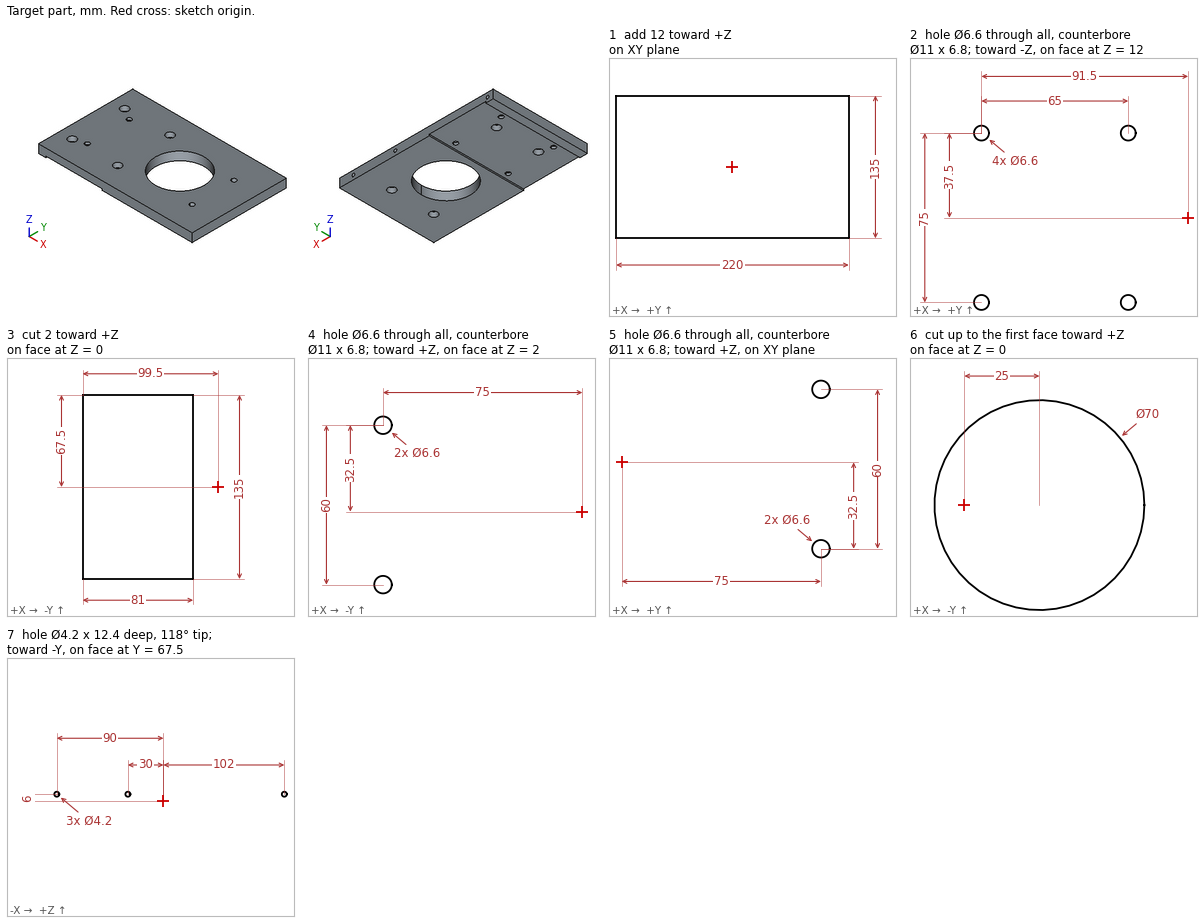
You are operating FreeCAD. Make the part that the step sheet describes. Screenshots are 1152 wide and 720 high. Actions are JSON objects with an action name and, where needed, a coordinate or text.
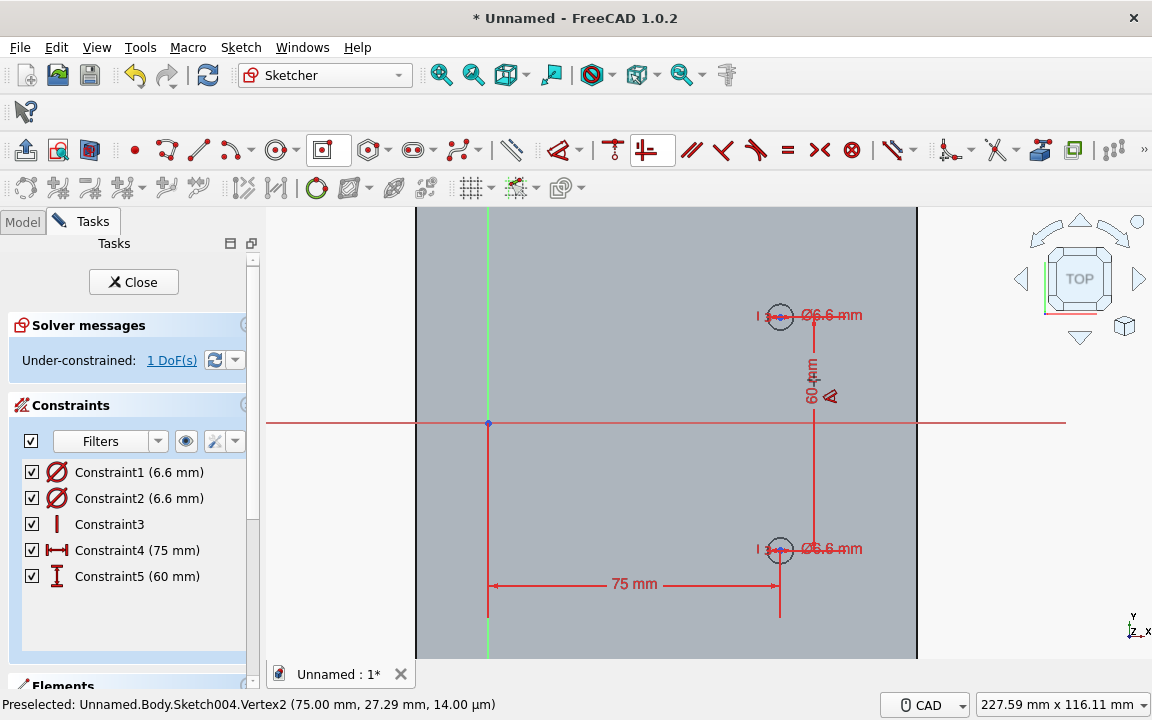
{"action": "left_click", "coordinate": [780, 551]}
{"action": "left_click", "coordinate": [454, 487]}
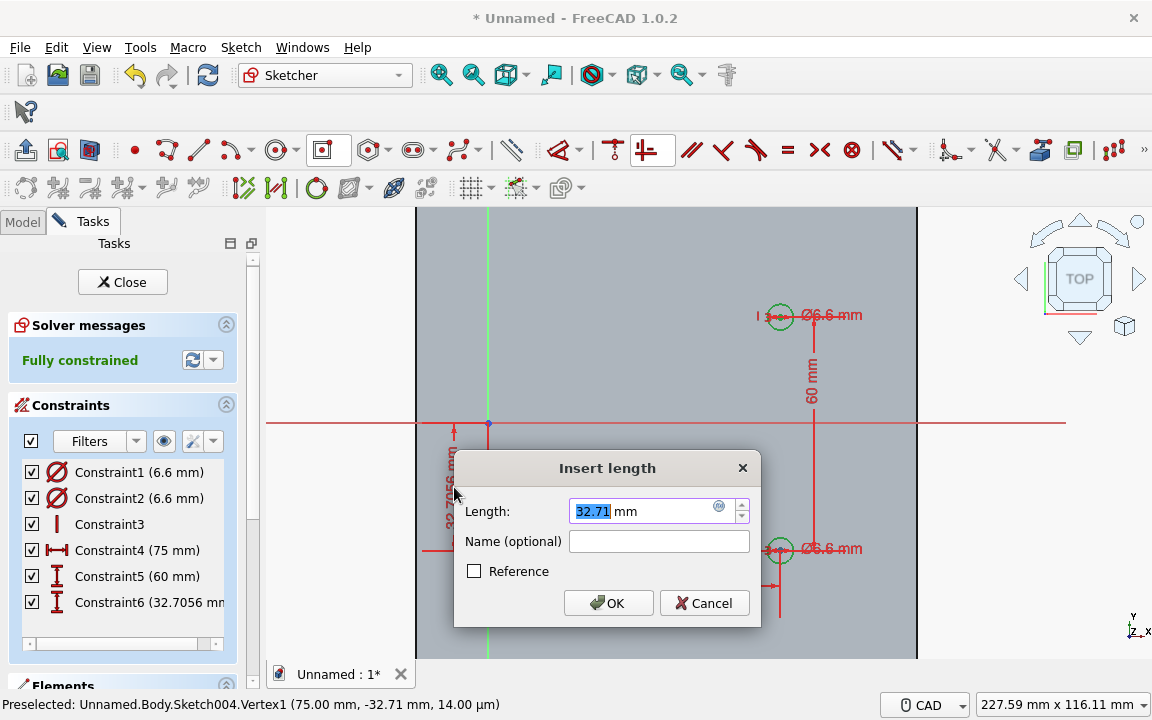
{"action": "type", "text": "32.5"}
{"action": "key", "text": "Return"}
{"action": "key", "text": "Escape"}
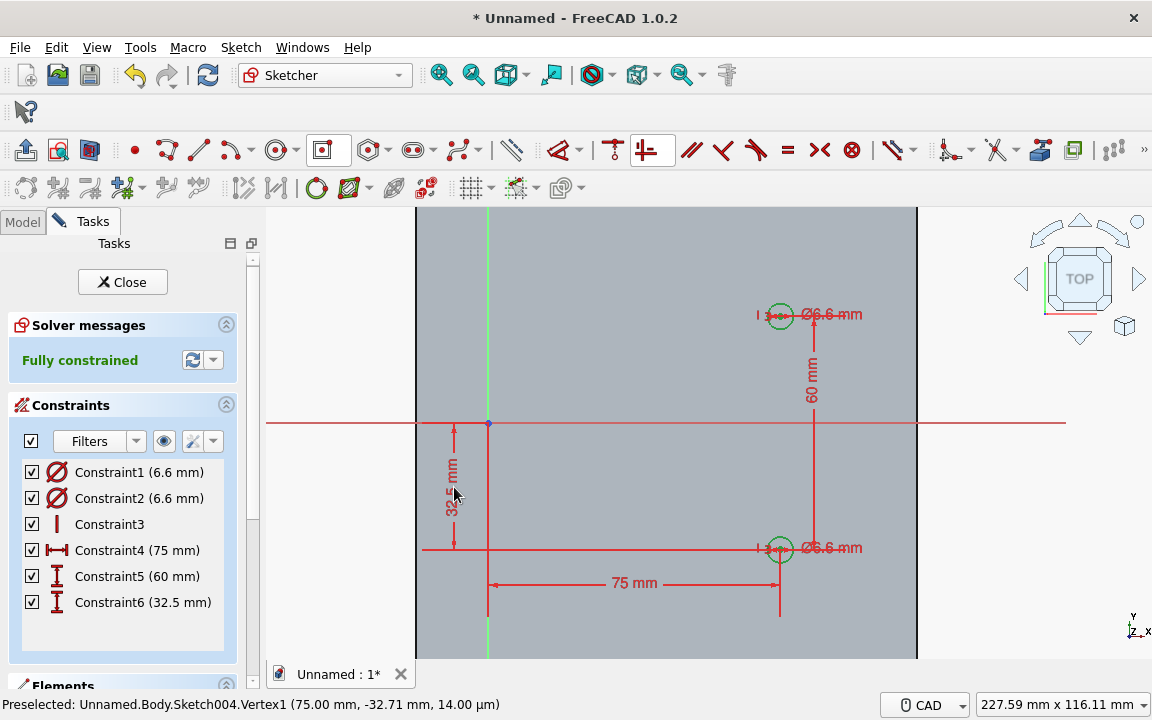
{"action": "left_click", "coordinate": [123, 282]}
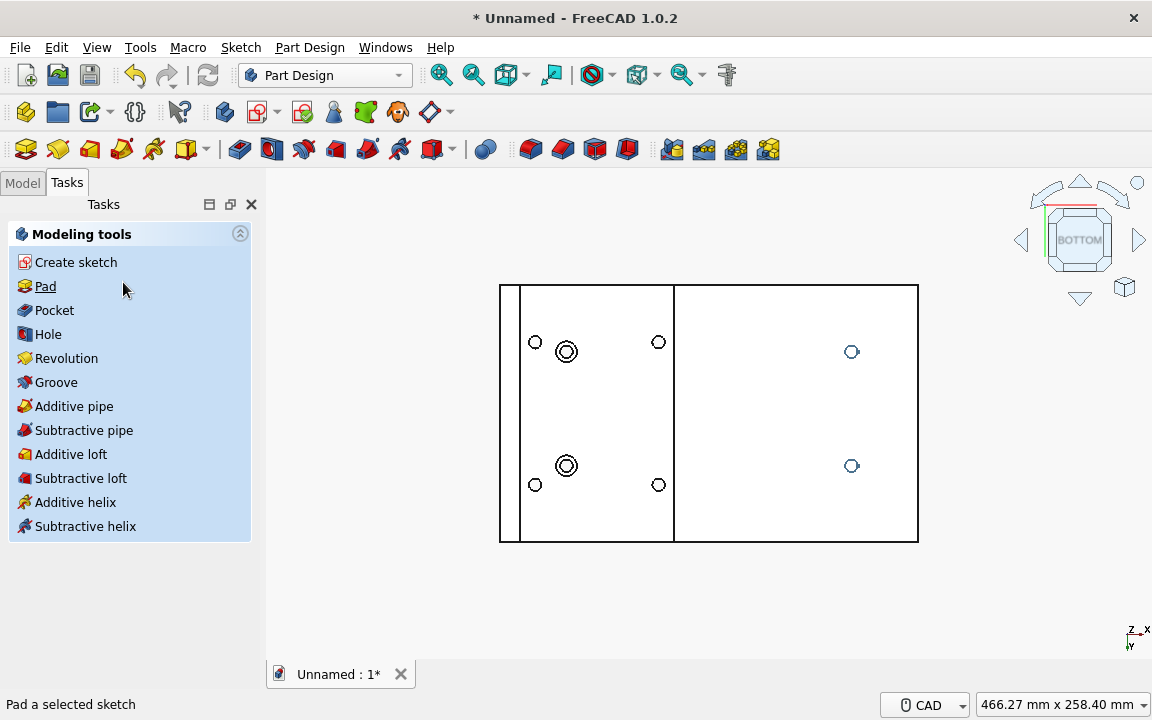
{"action": "left_click", "coordinate": [272, 150]}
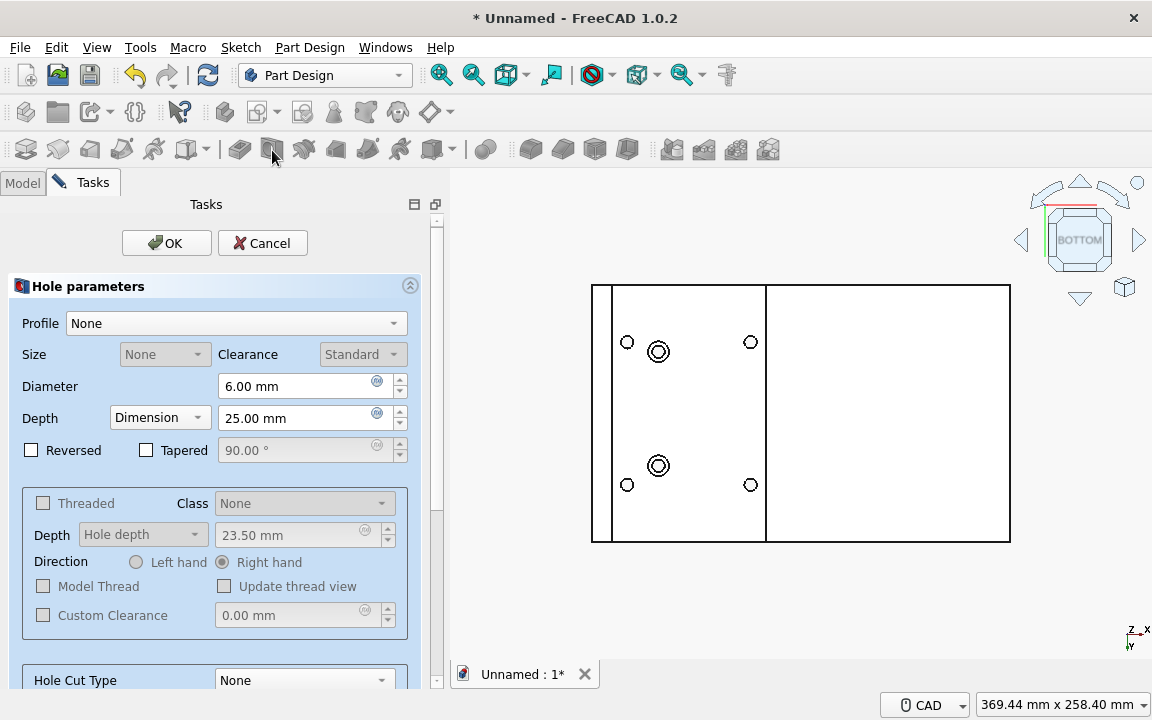
{"action": "triple_click", "coordinate": [305, 386]}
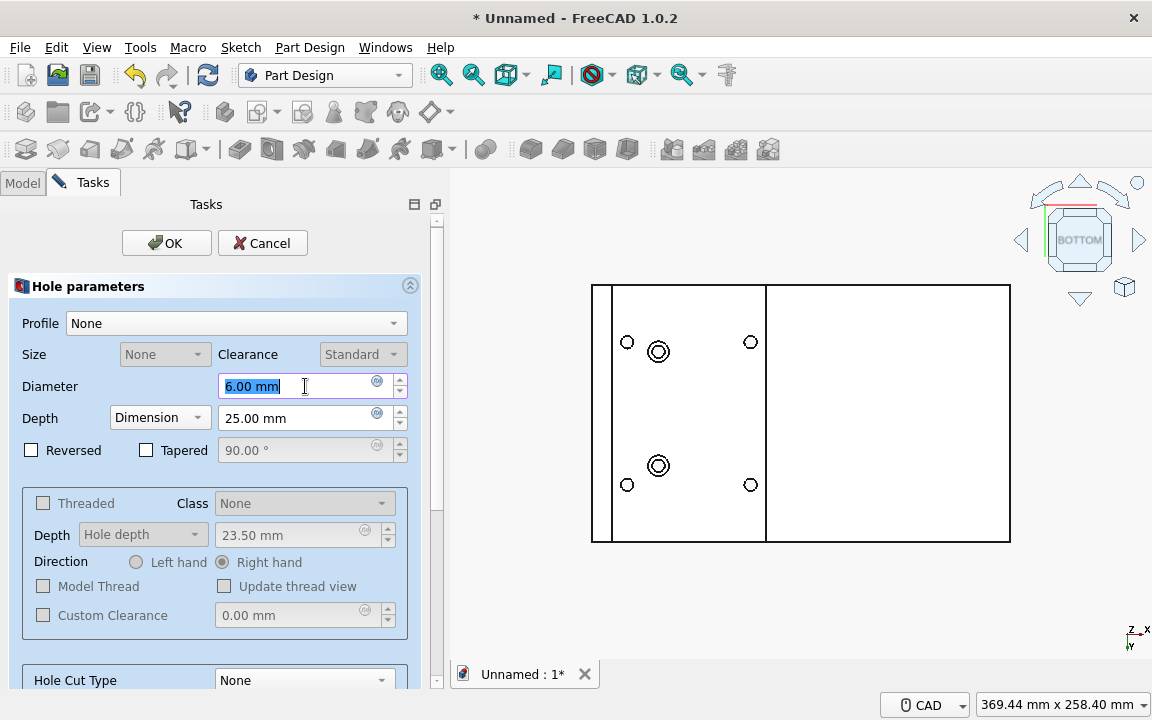
{"action": "type", "text": "6.6"}
{"action": "key", "text": "Tab"}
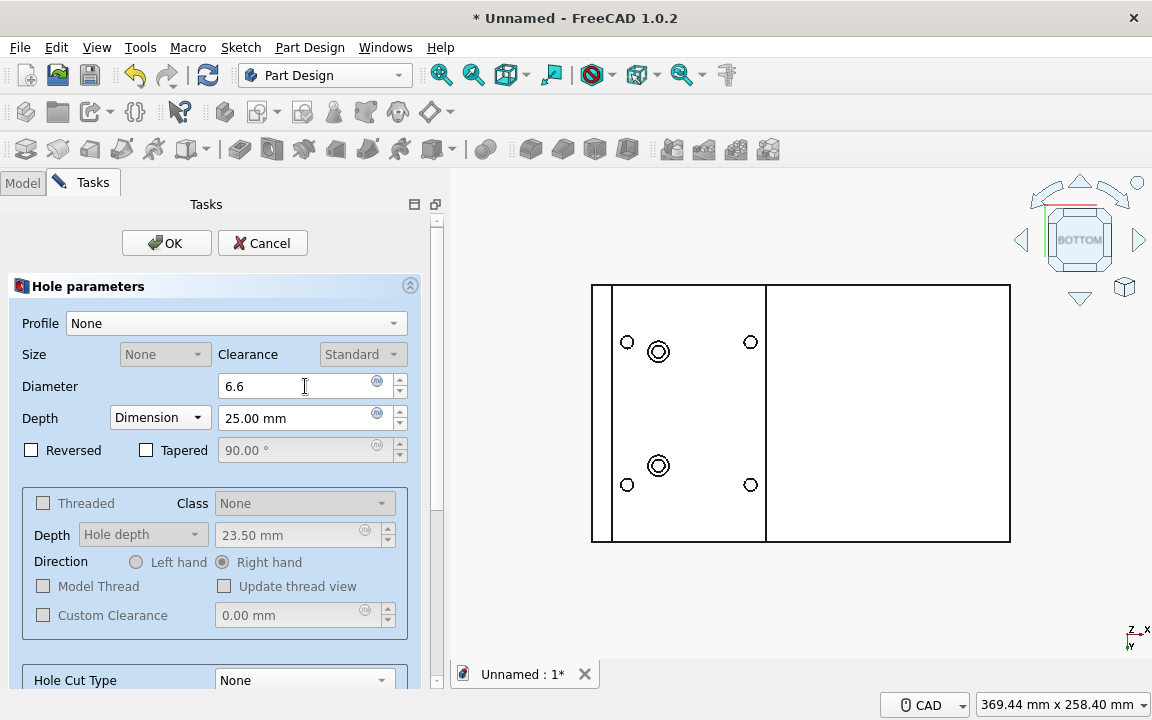
{"action": "left_click", "coordinate": [161, 418]}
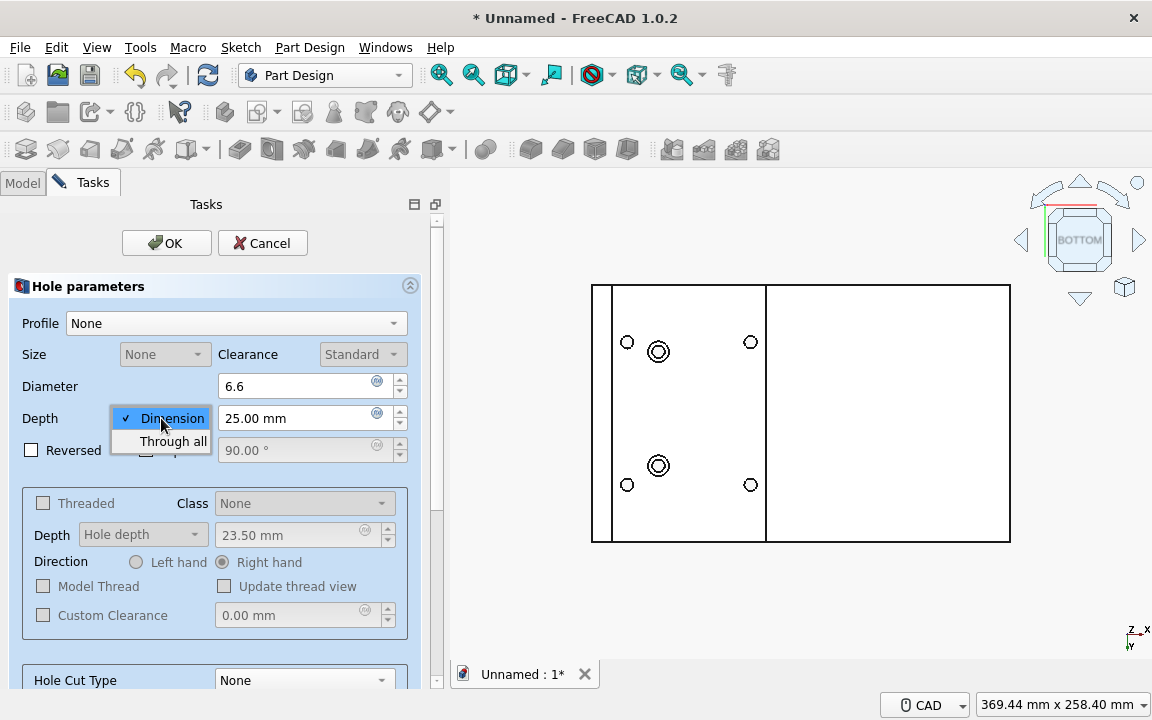
{"action": "left_click", "coordinate": [160, 442]}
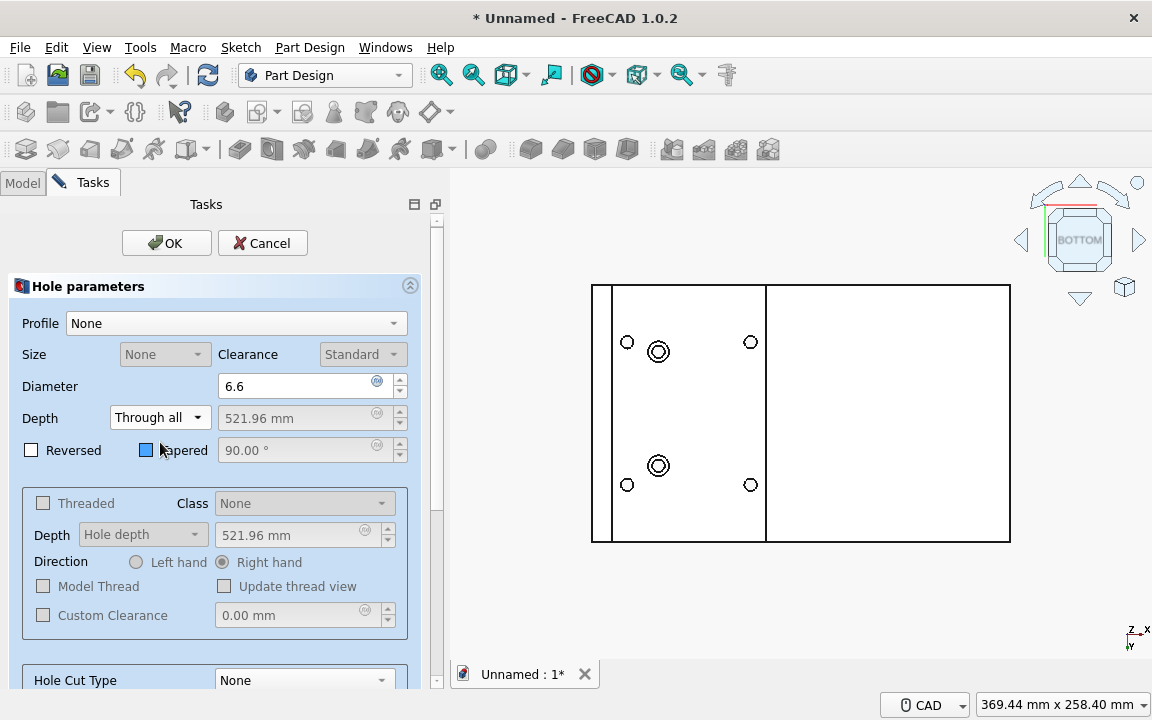
{"action": "left_click", "coordinate": [30, 450]}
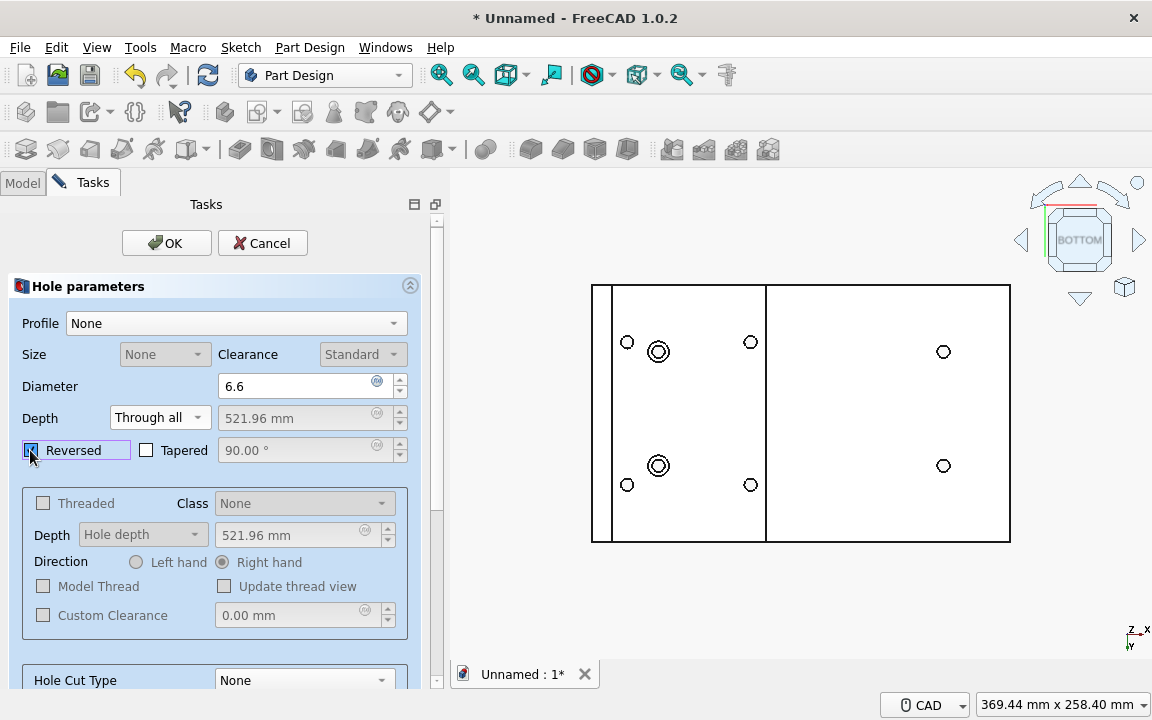
{"action": "scroll", "coordinate": [437, 451], "scroll_direction": "down", "scroll_amount": 2}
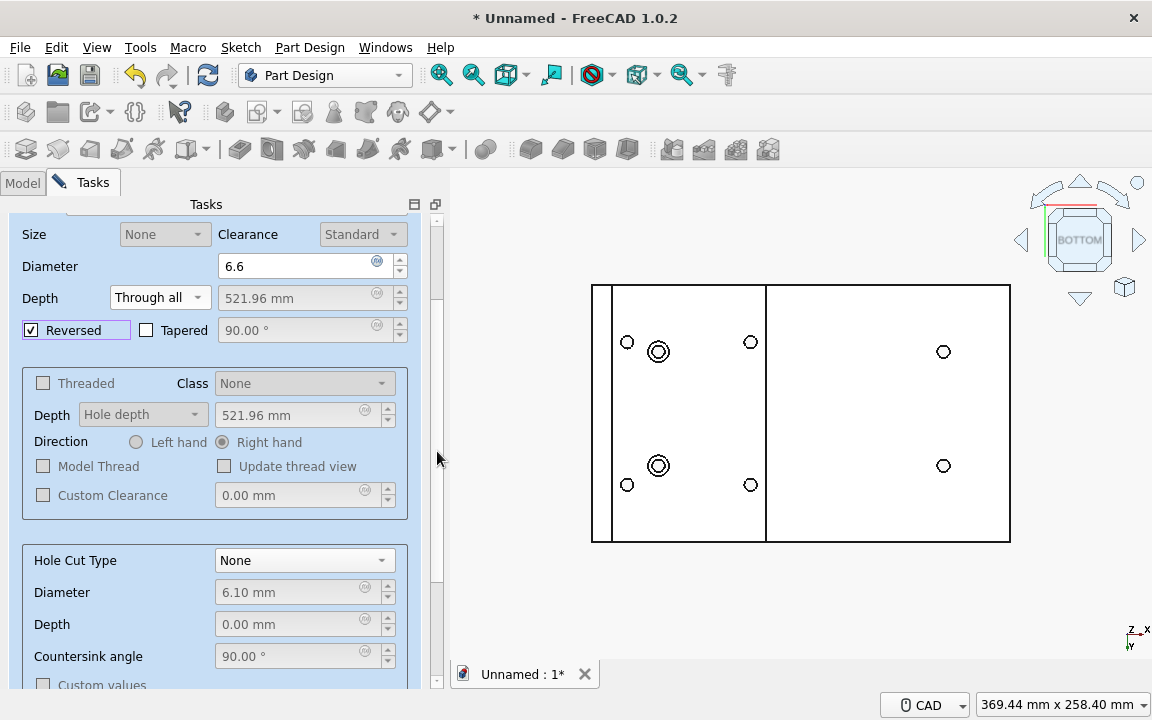
{"action": "left_click", "coordinate": [306, 560]}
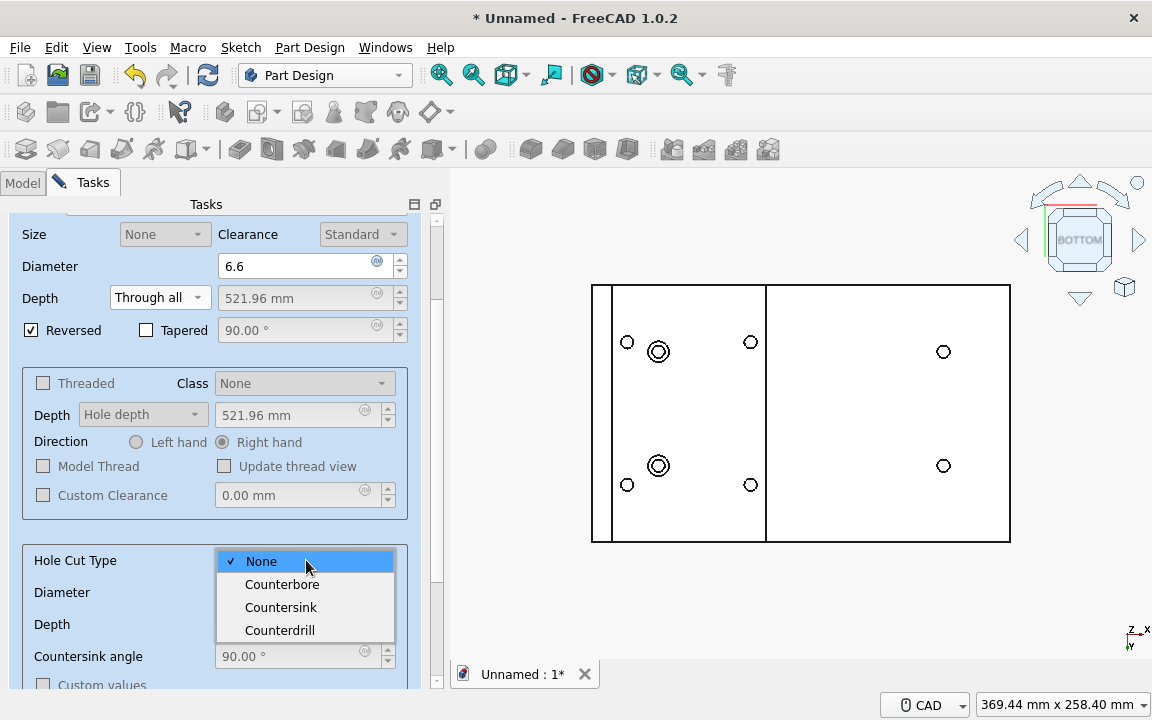
{"action": "left_click", "coordinate": [304, 584]}